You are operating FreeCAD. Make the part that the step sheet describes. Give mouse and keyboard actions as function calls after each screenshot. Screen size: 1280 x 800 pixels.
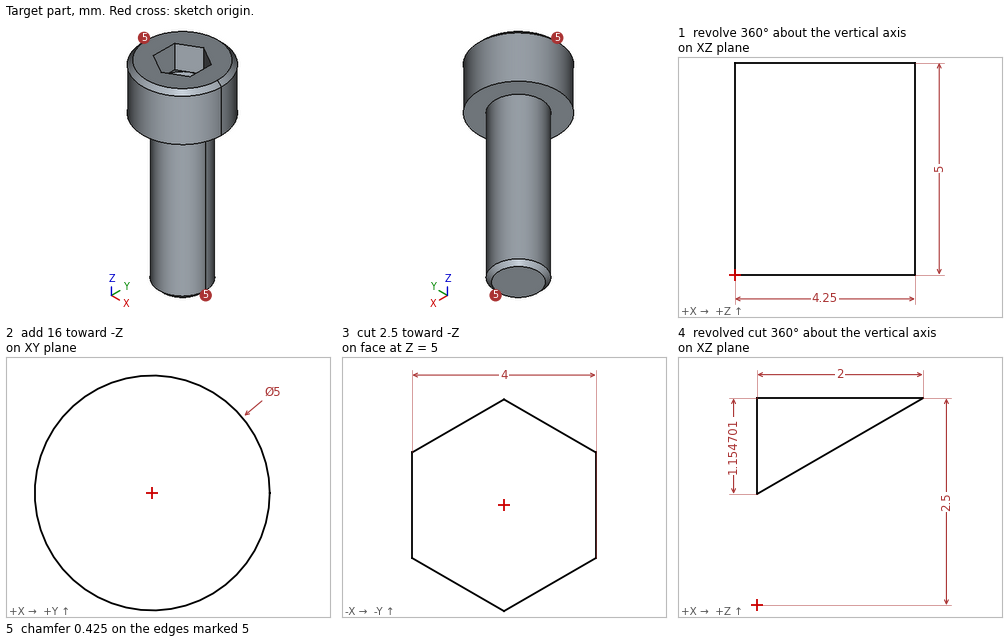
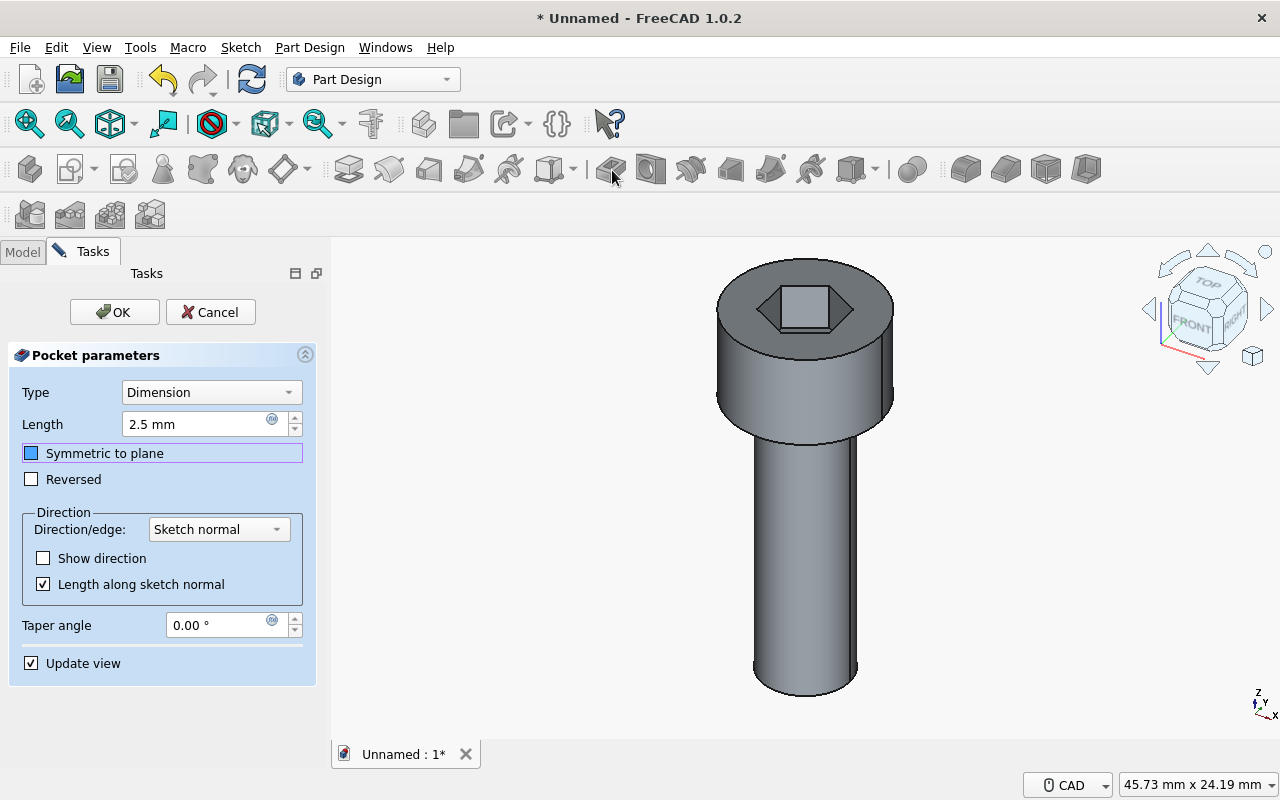
click(115, 312)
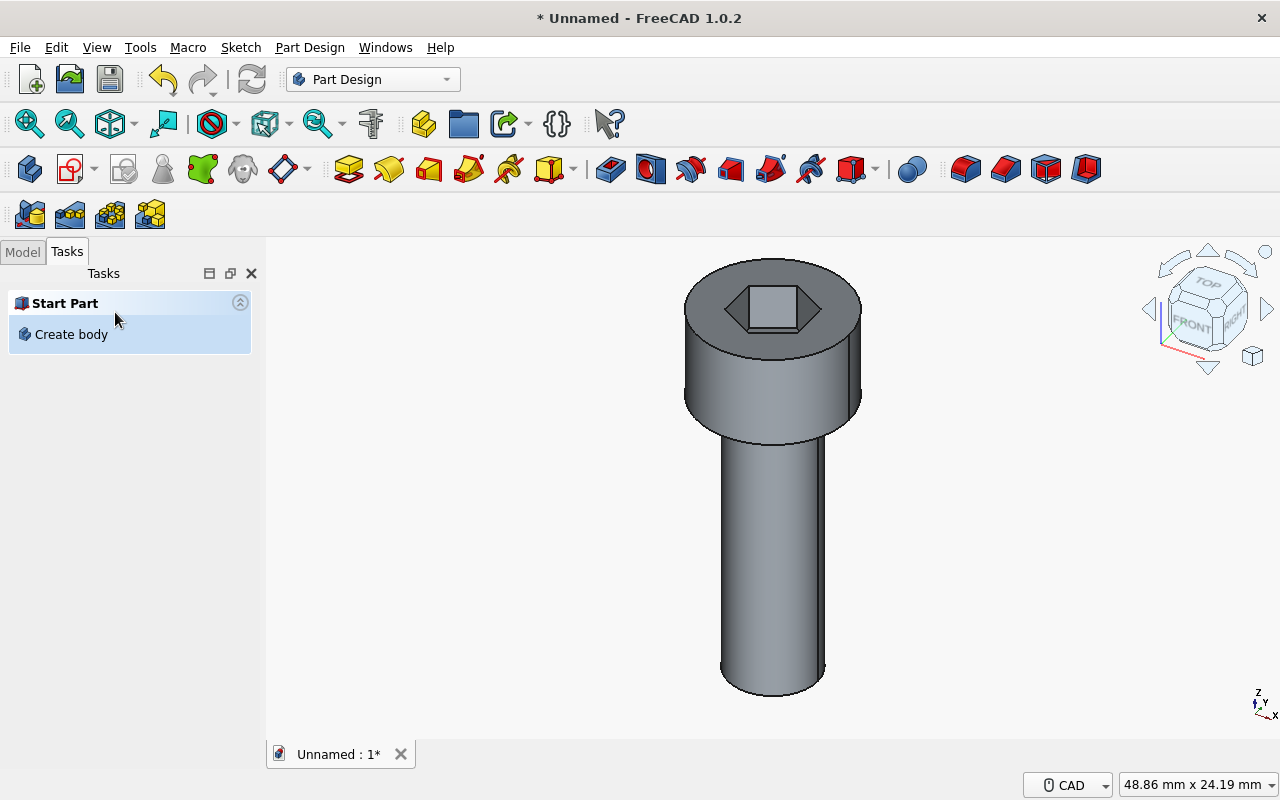
click(70, 170)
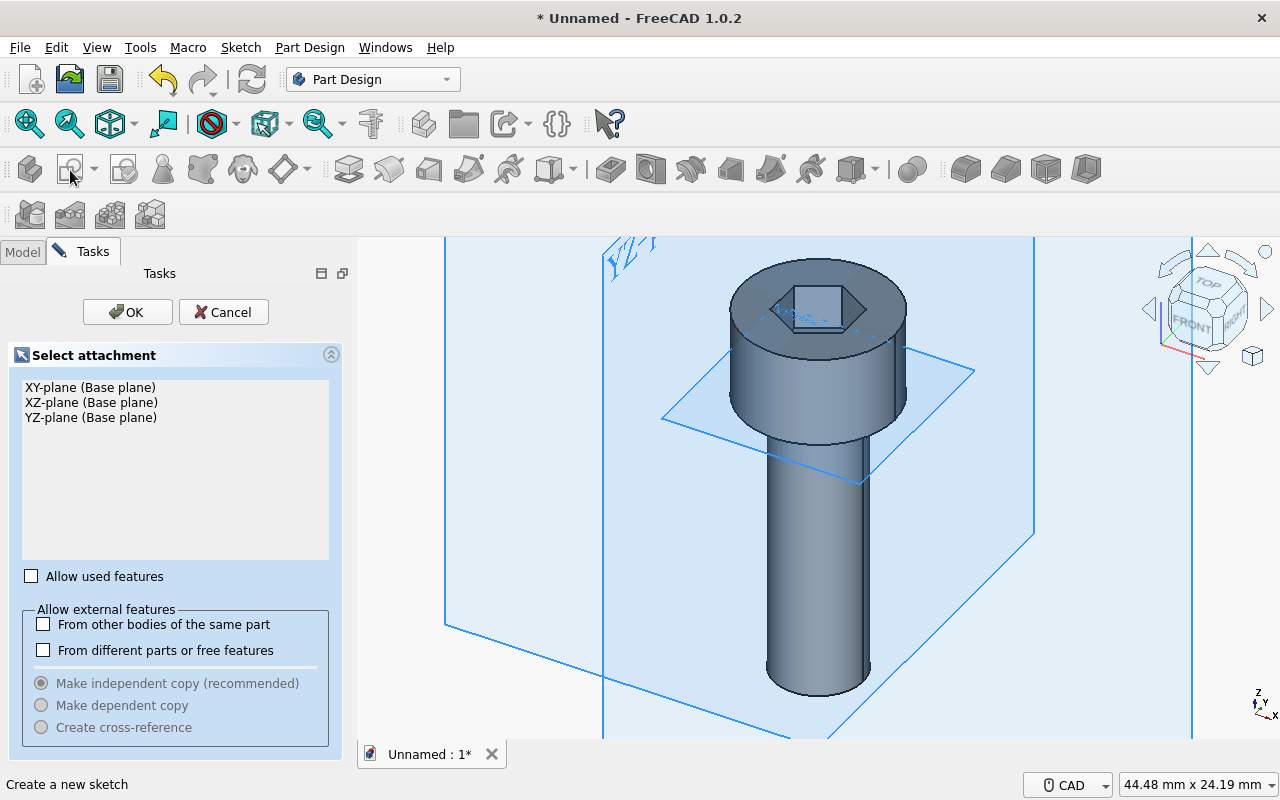
click(82, 402)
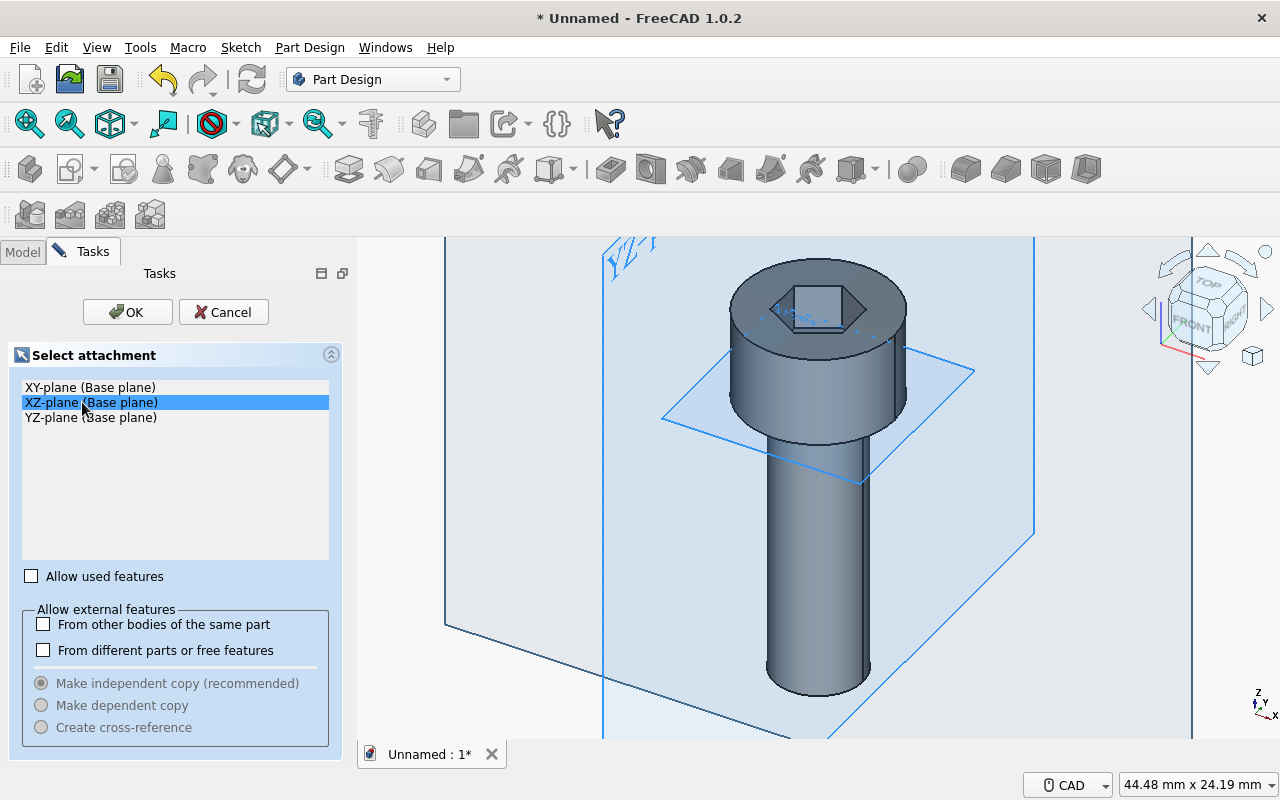
click(128, 312)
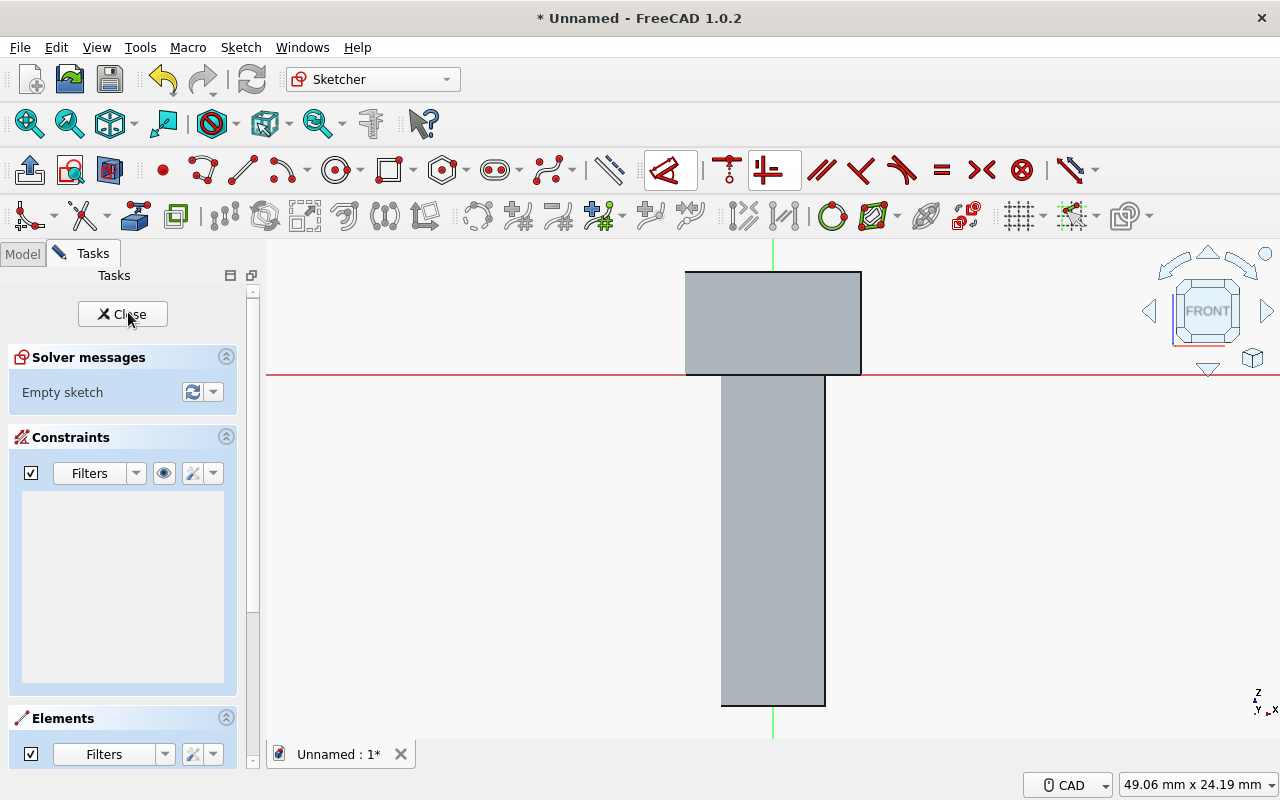
click(110, 170)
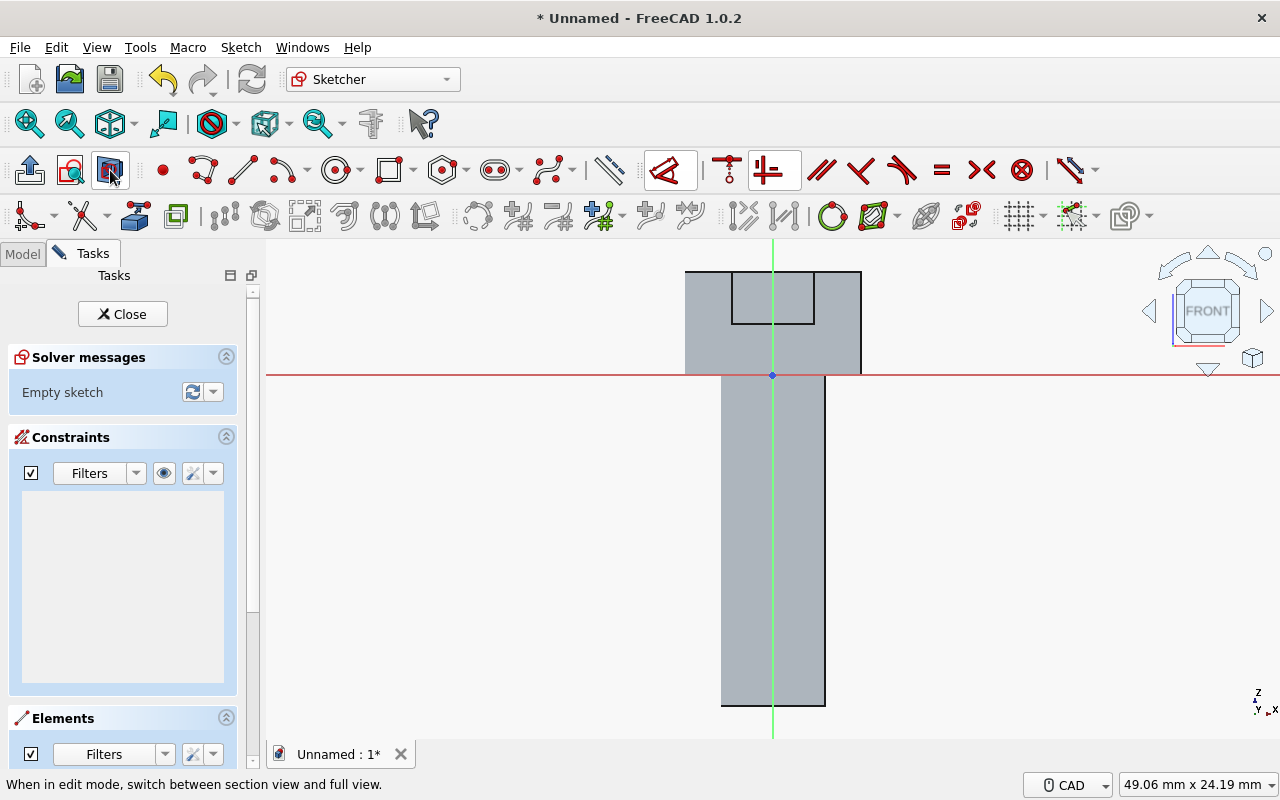
scroll(811, 322, up, 9)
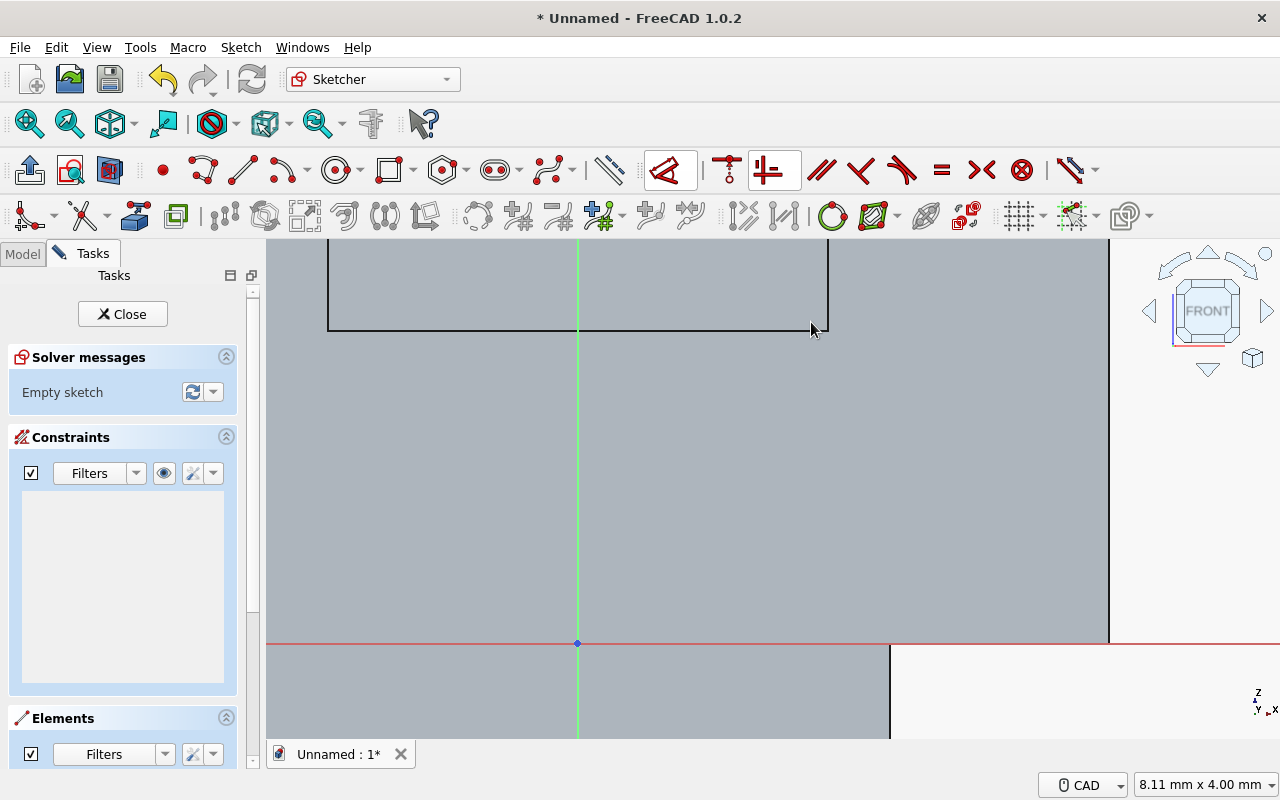
click(204, 170)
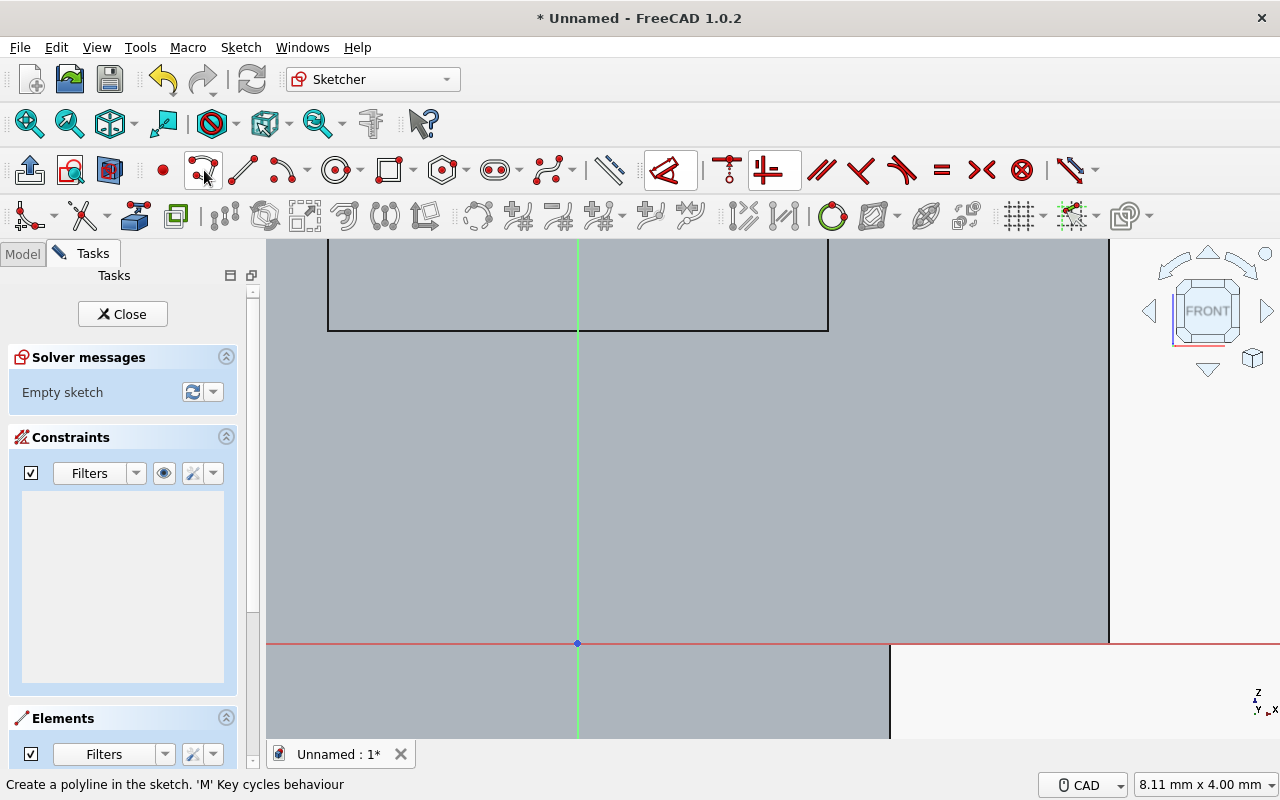
click(578, 476)
click(828, 331)
click(587, 331)
click(578, 477)
key(Escape)
key(Escape)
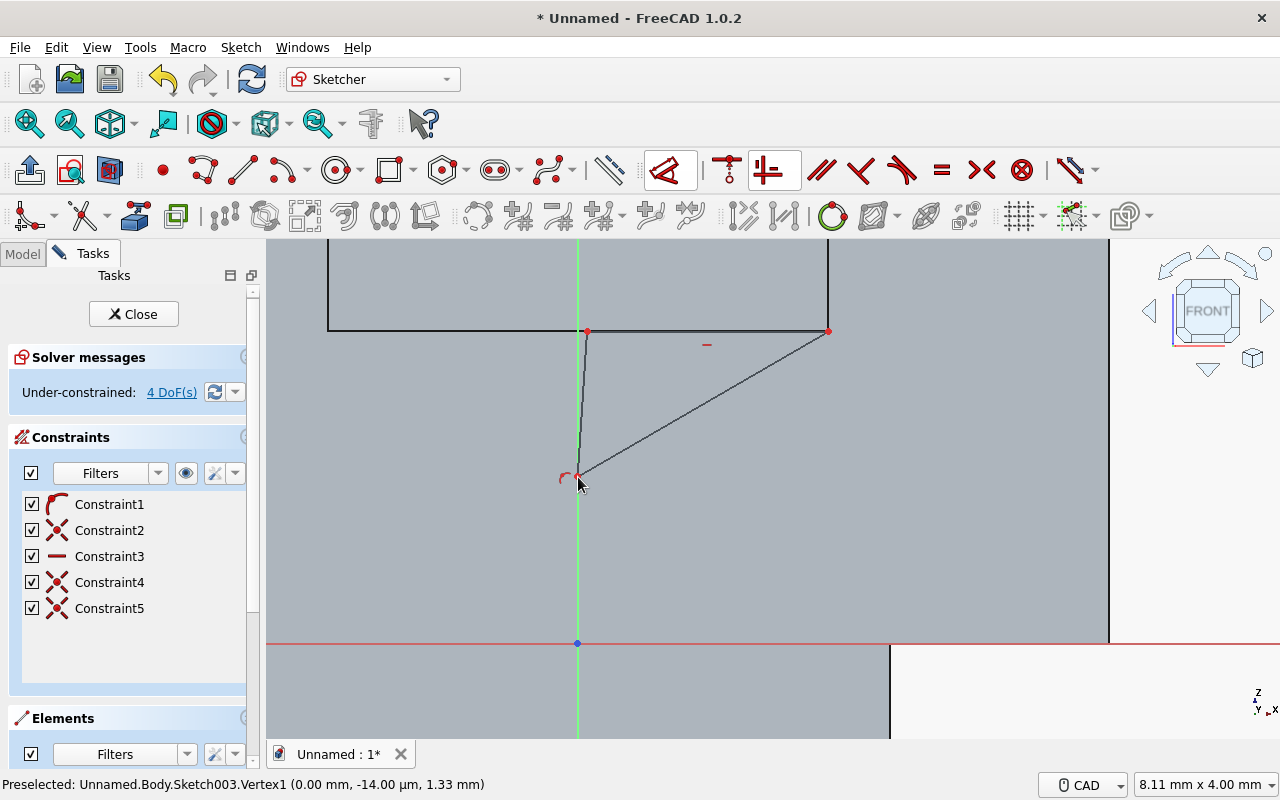
click(580, 434)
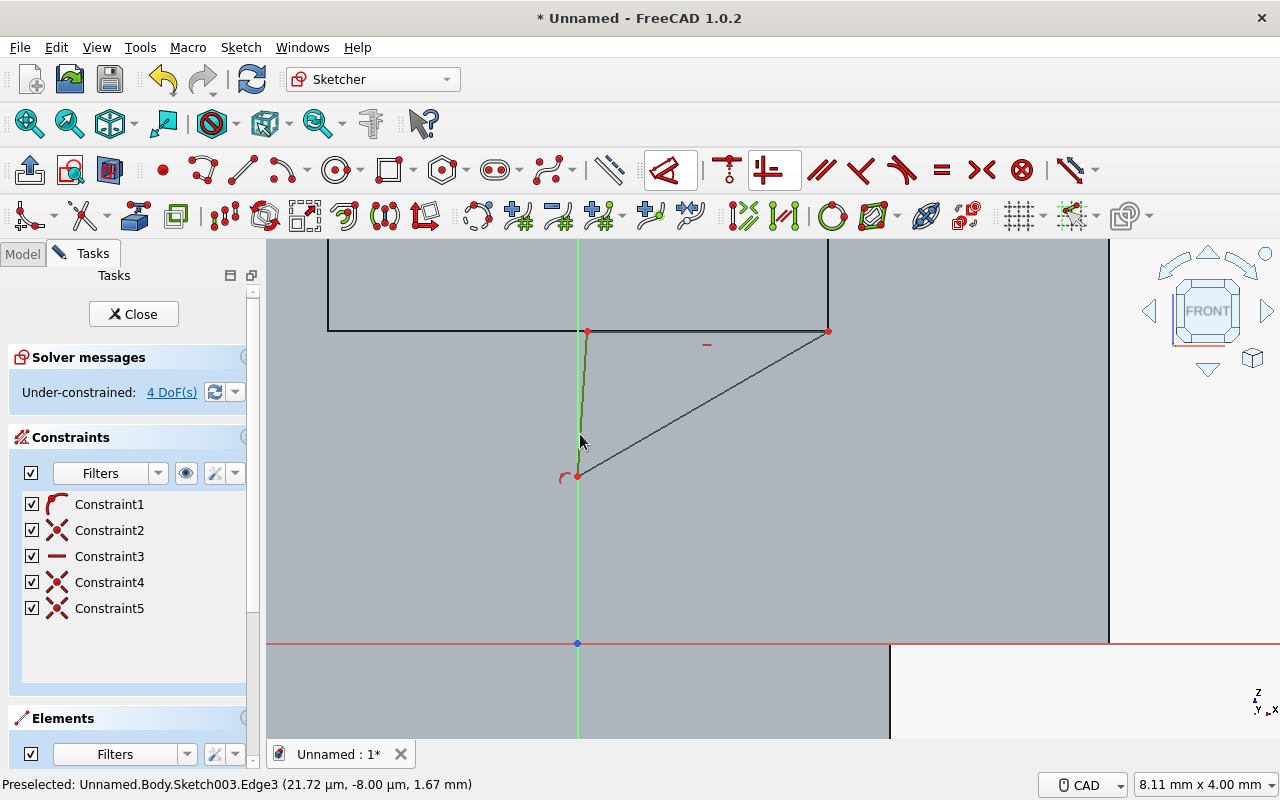
key(v)